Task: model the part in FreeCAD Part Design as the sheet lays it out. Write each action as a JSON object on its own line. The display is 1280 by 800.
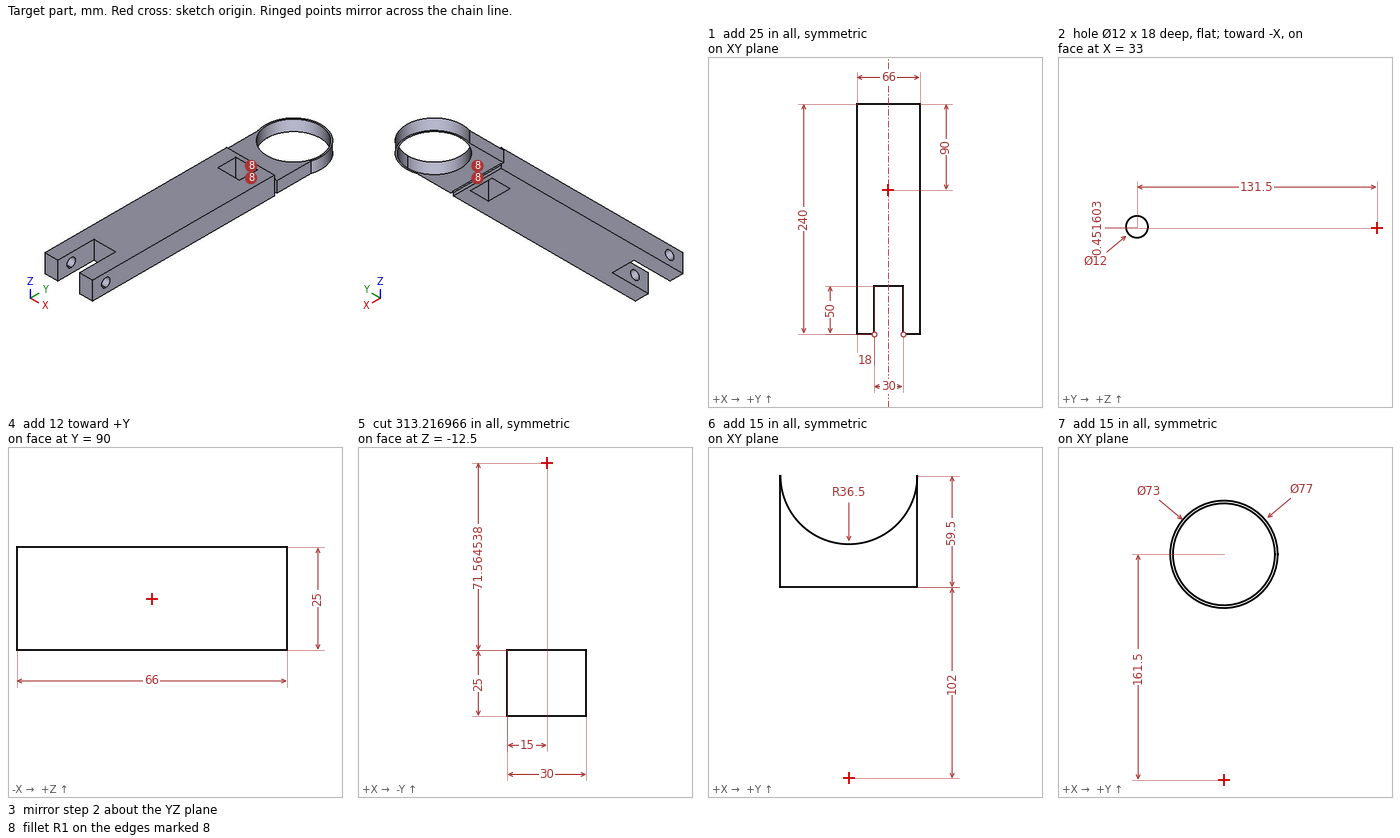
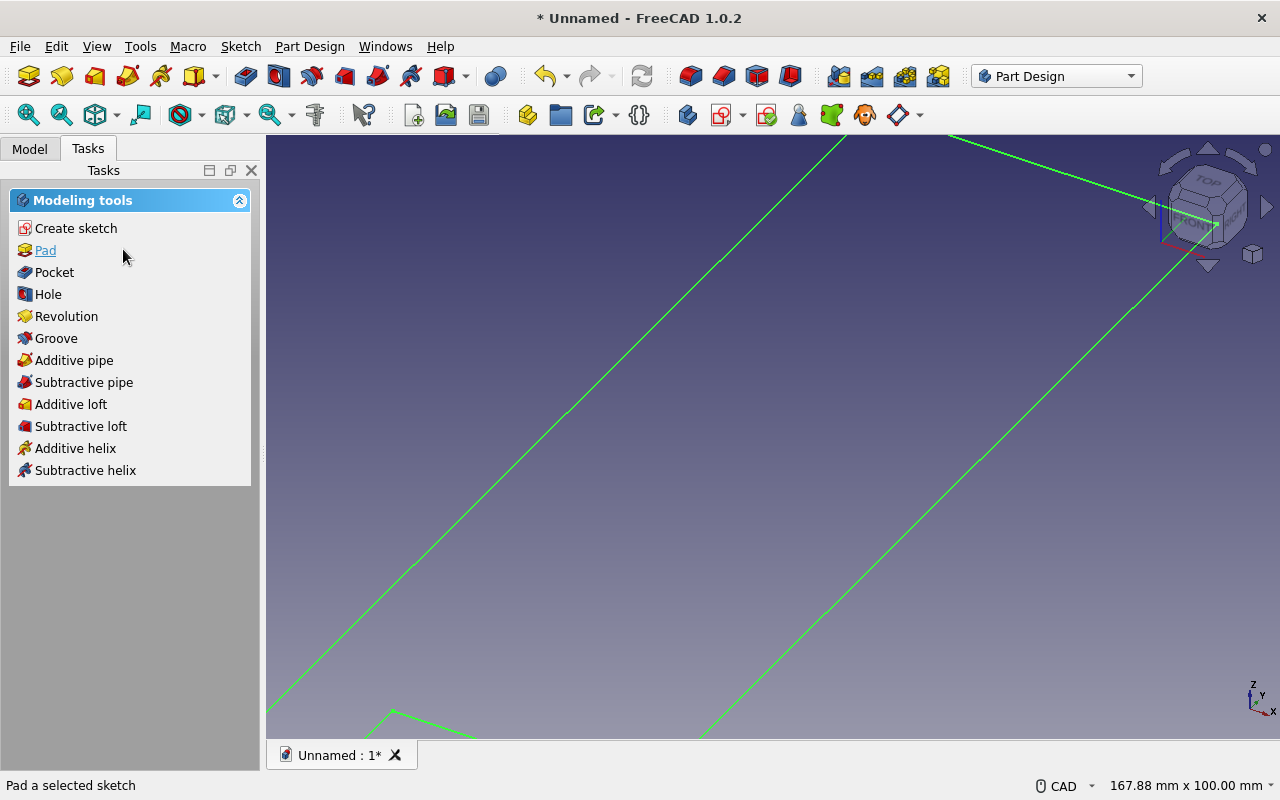
{"action": "left_click", "coordinate": [29, 76]}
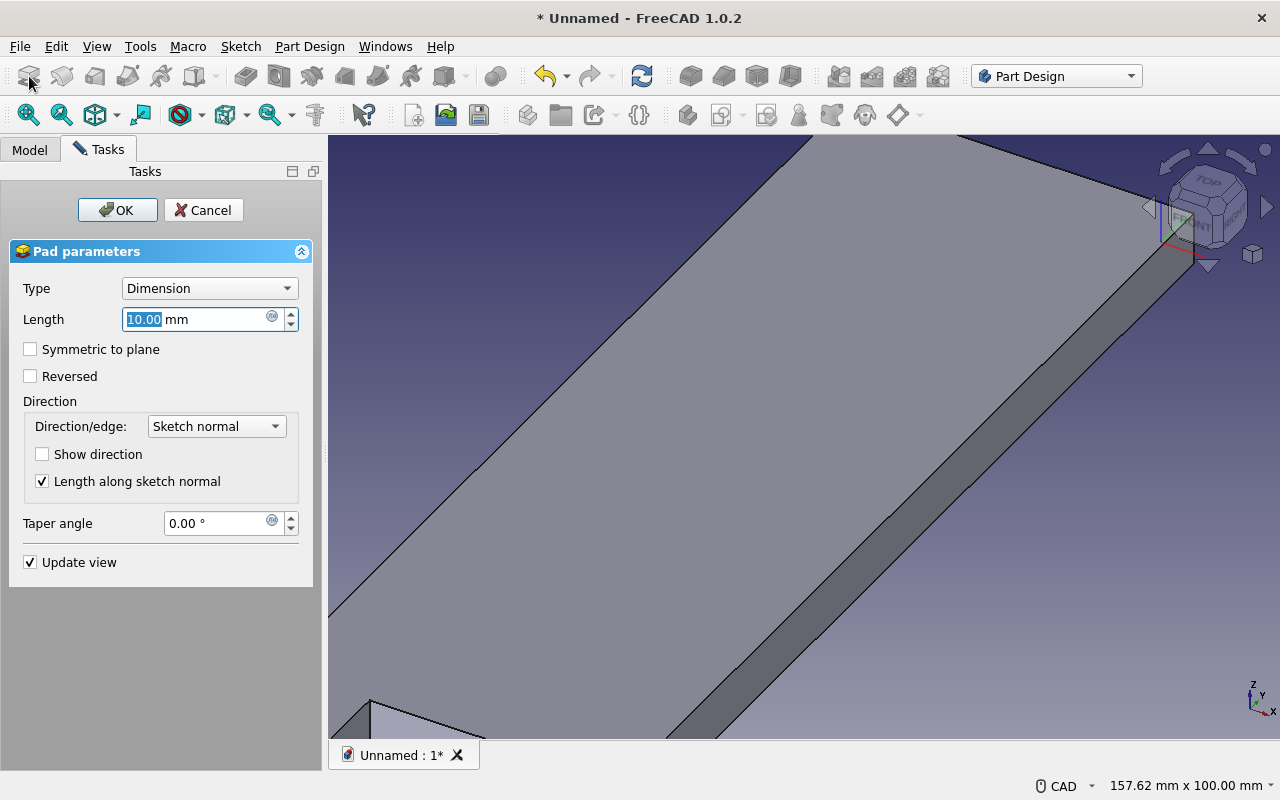
{"action": "type", "text": "25"}
{"action": "key", "text": "Tab"}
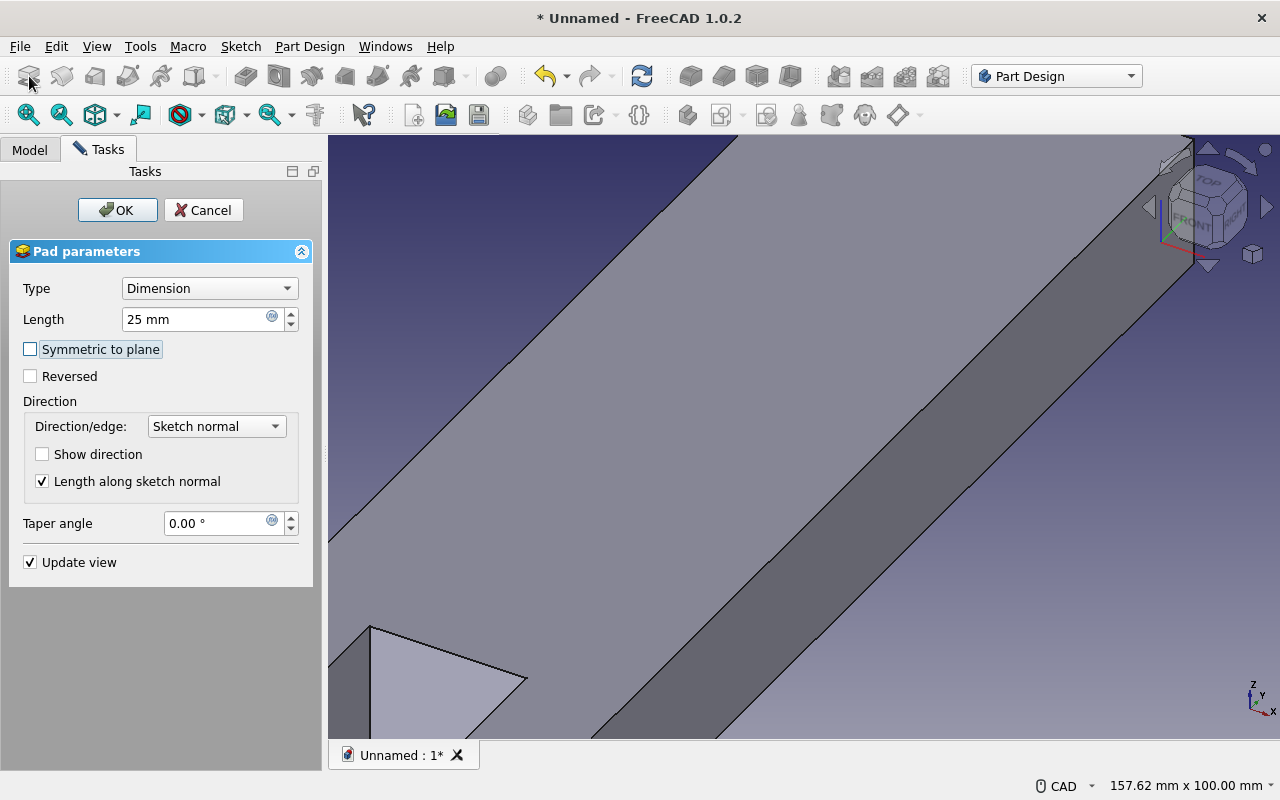
{"action": "left_click", "coordinate": [31, 349]}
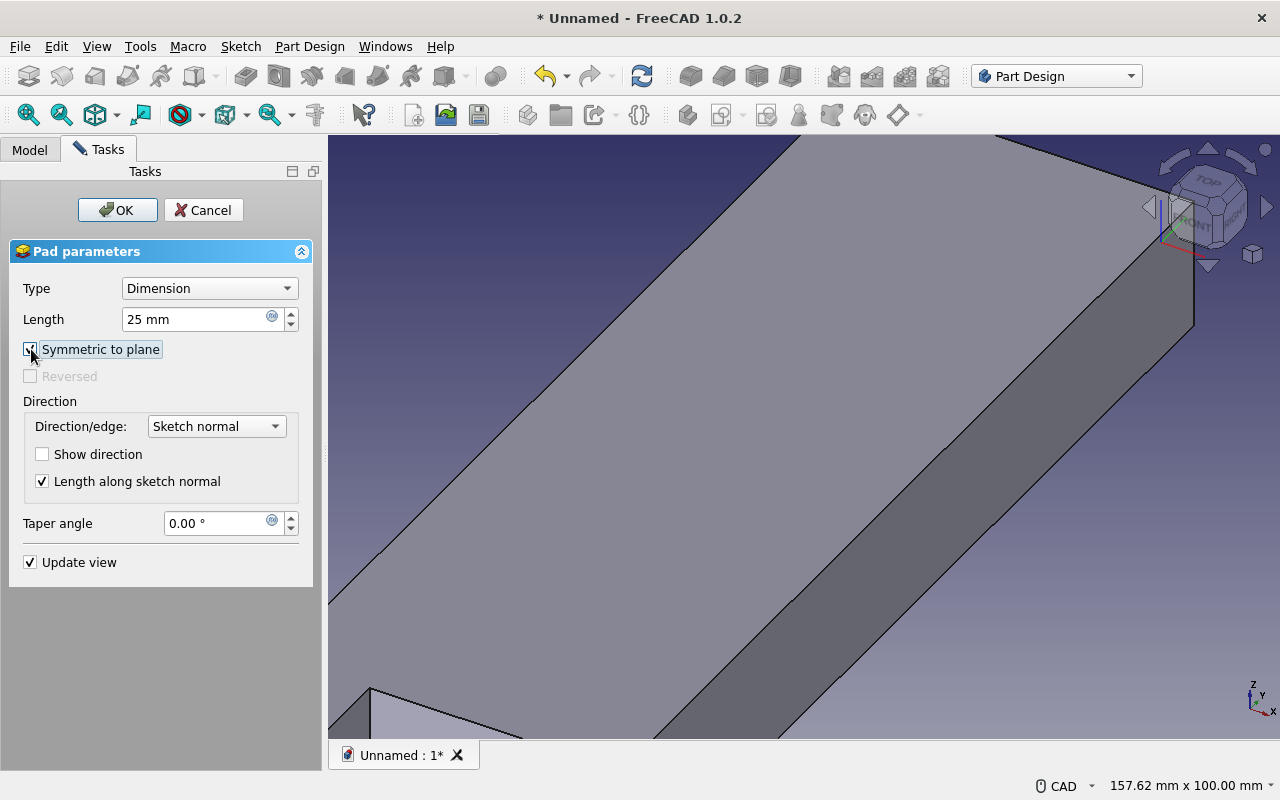
{"action": "left_click", "coordinate": [118, 210]}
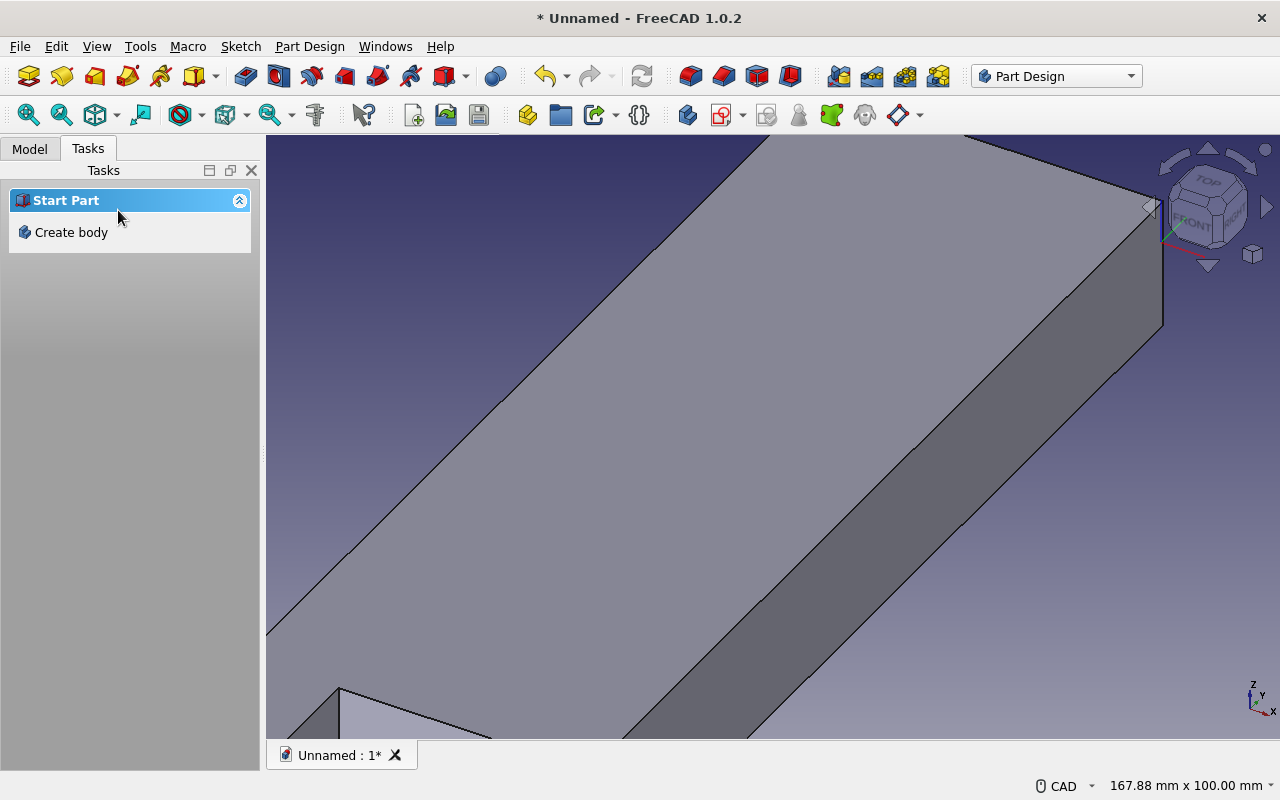
{"action": "key", "text": "v f"}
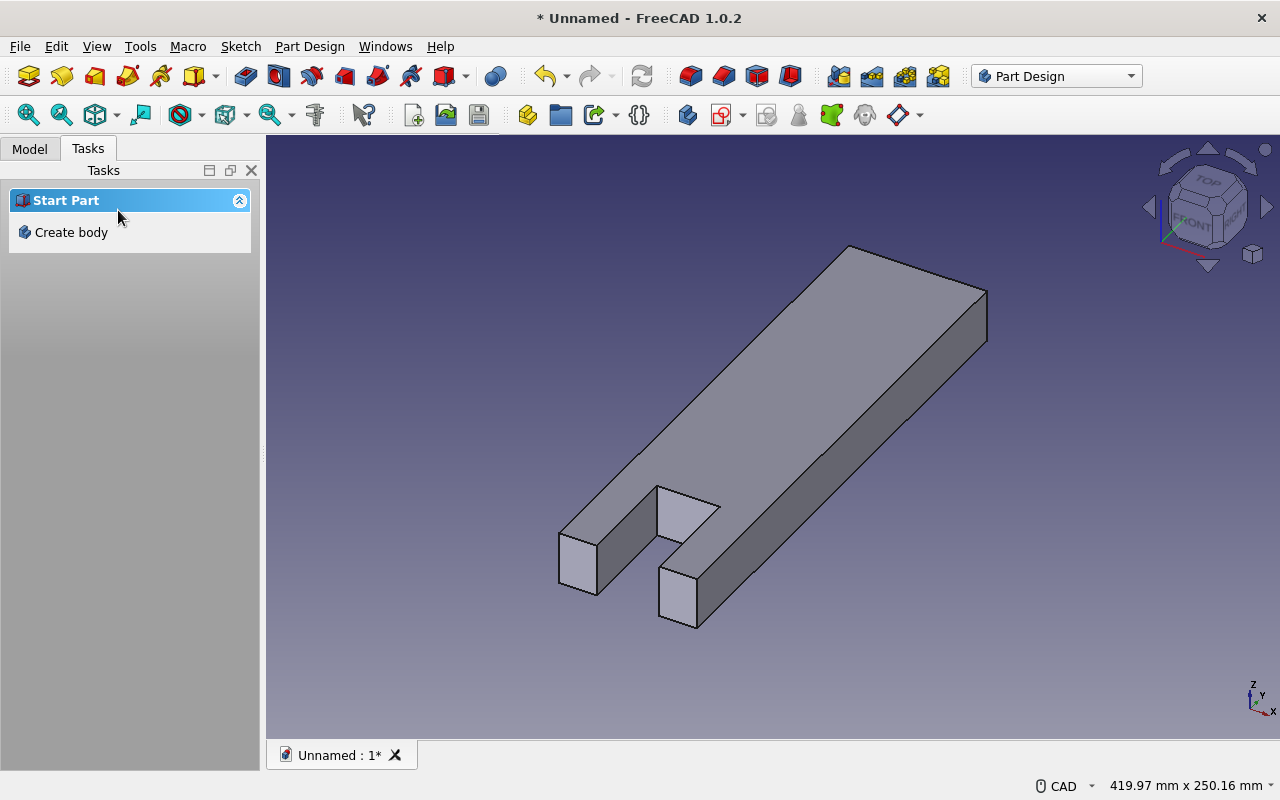
{"action": "left_click", "coordinate": [966, 335]}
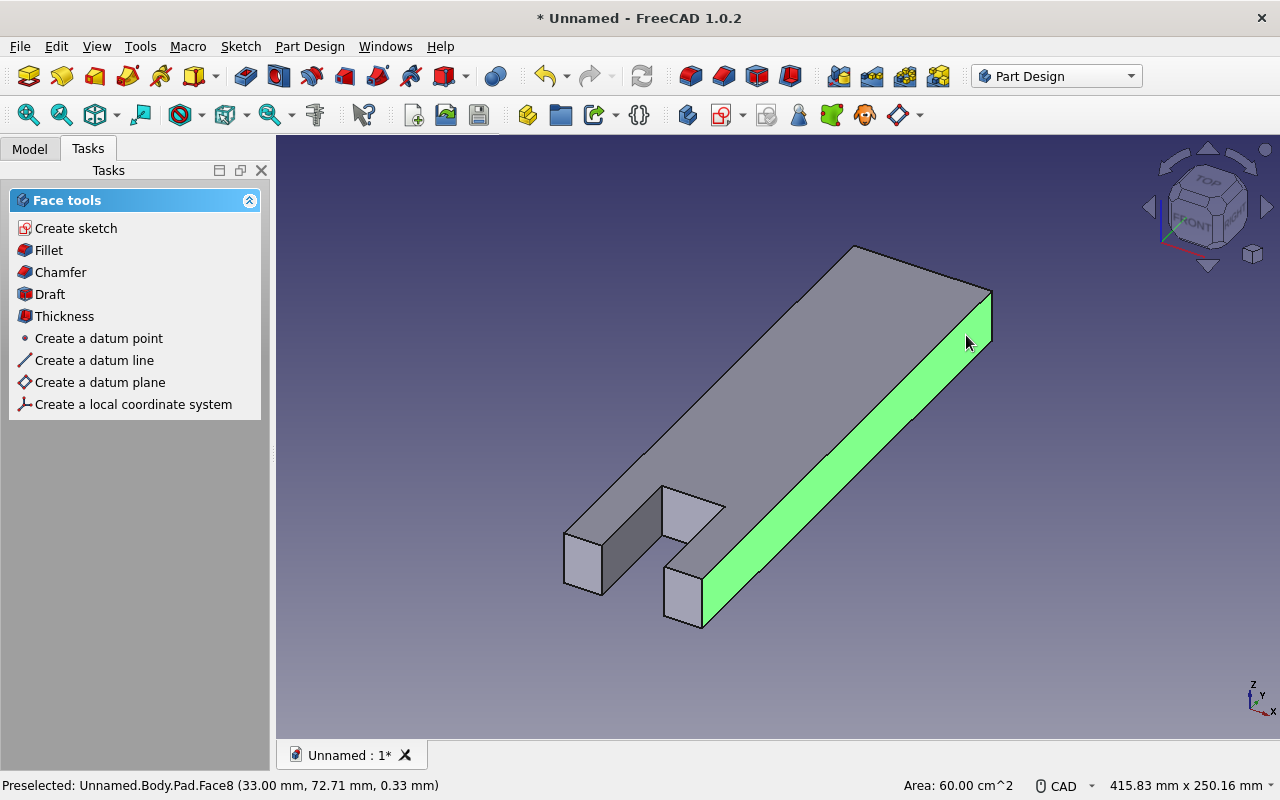
{"action": "left_click", "coordinate": [720, 116]}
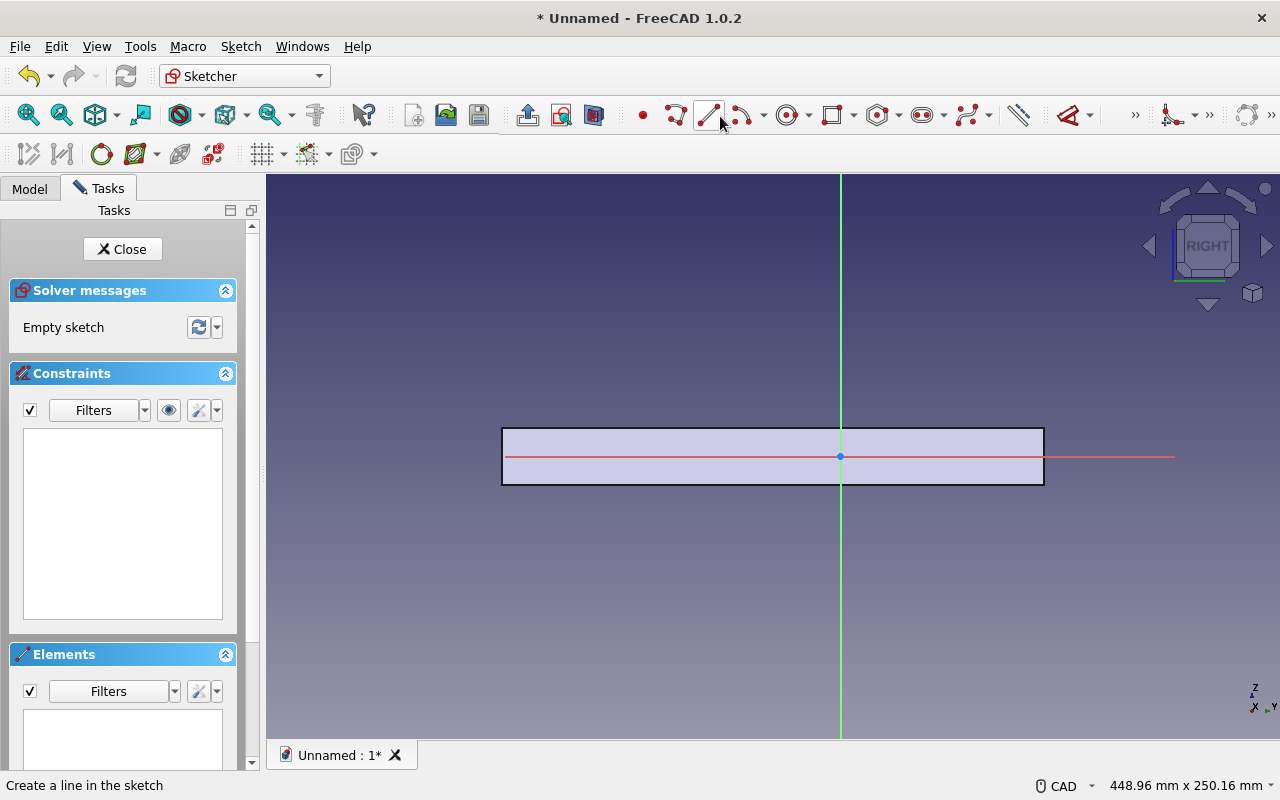
{"action": "scroll", "coordinate": [531, 455], "scroll_direction": "up", "scroll_amount": 13}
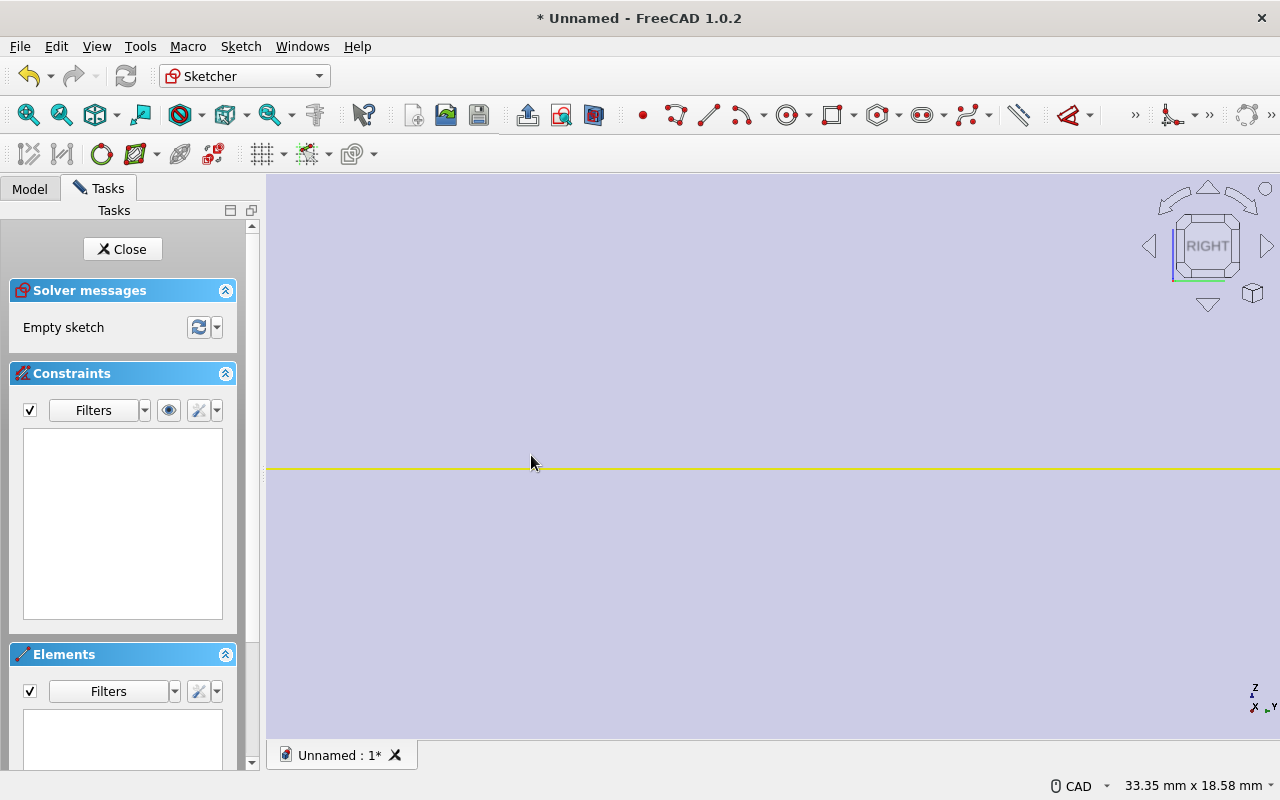
{"action": "left_click", "coordinate": [786, 116]}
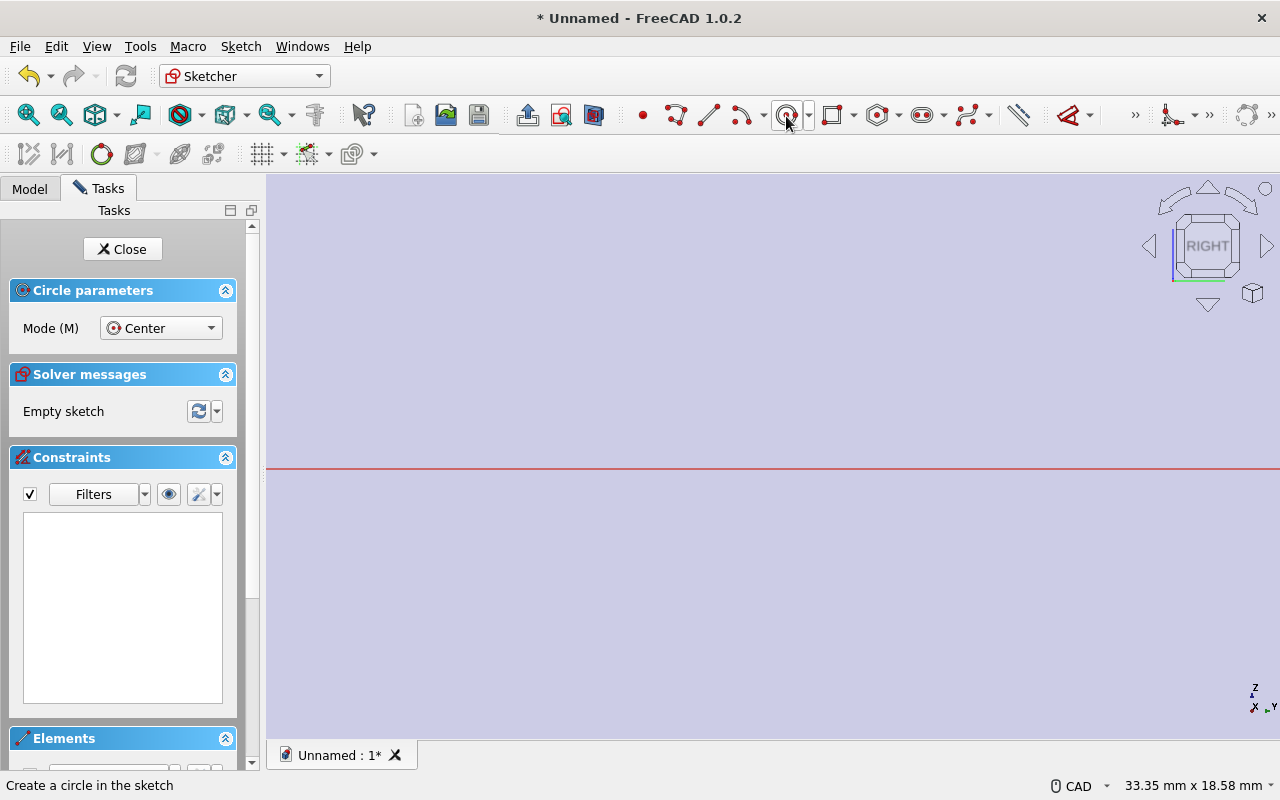
{"action": "left_click", "coordinate": [700, 455]}
{"action": "left_click", "coordinate": [829, 326]}
{"action": "key", "text": "Escape"}